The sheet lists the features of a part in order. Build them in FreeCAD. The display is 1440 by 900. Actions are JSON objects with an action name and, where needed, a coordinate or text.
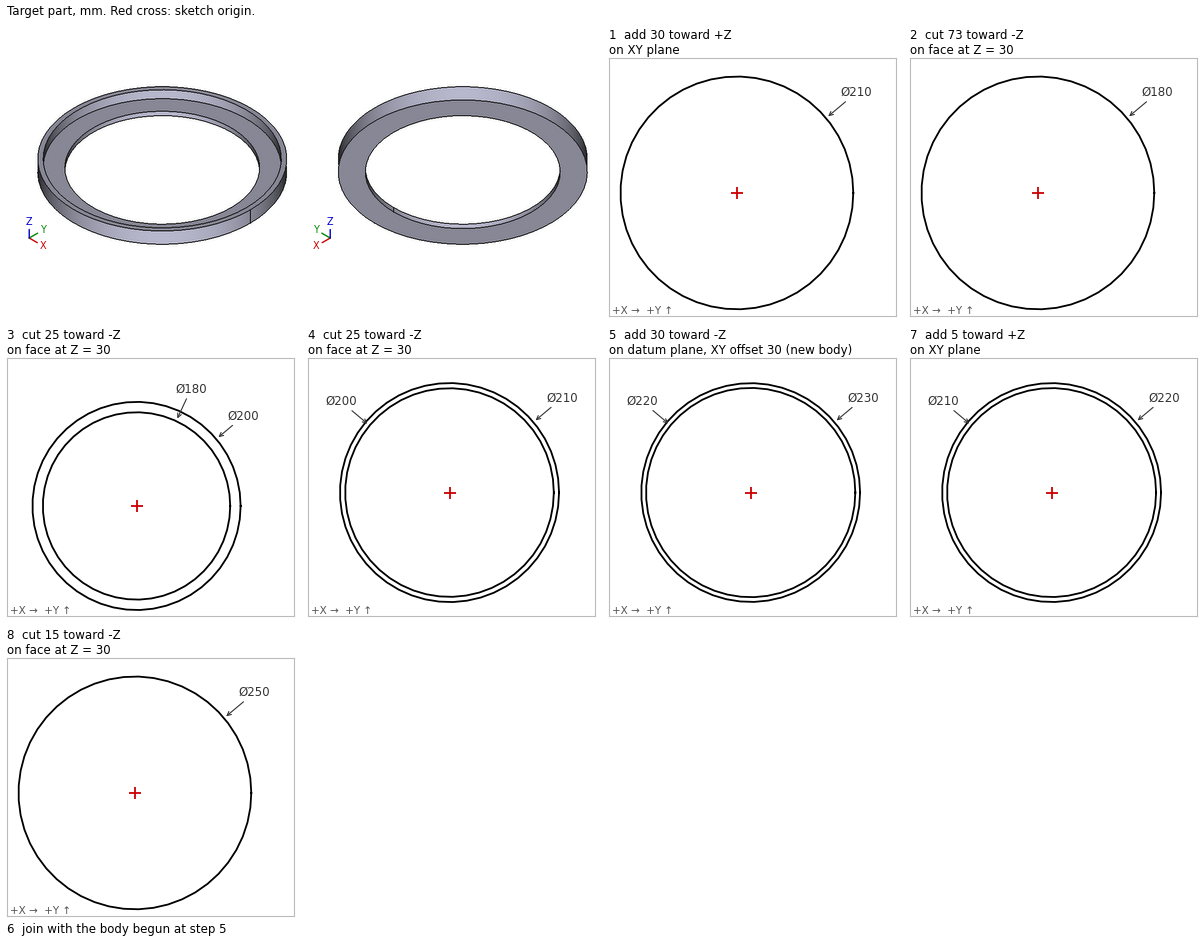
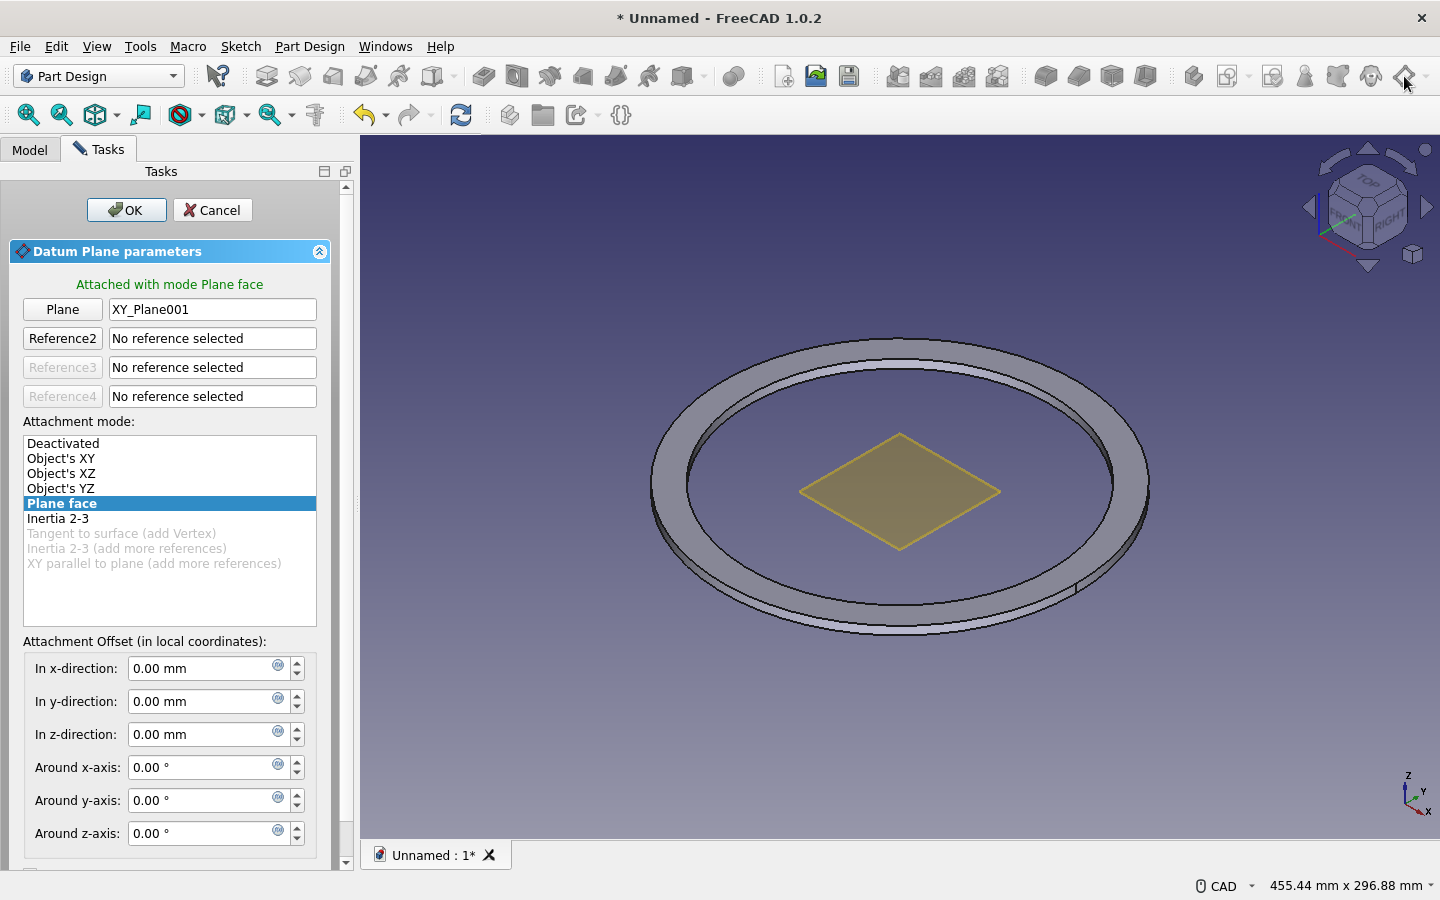
{"action": "triple_click", "coordinate": [210, 734]}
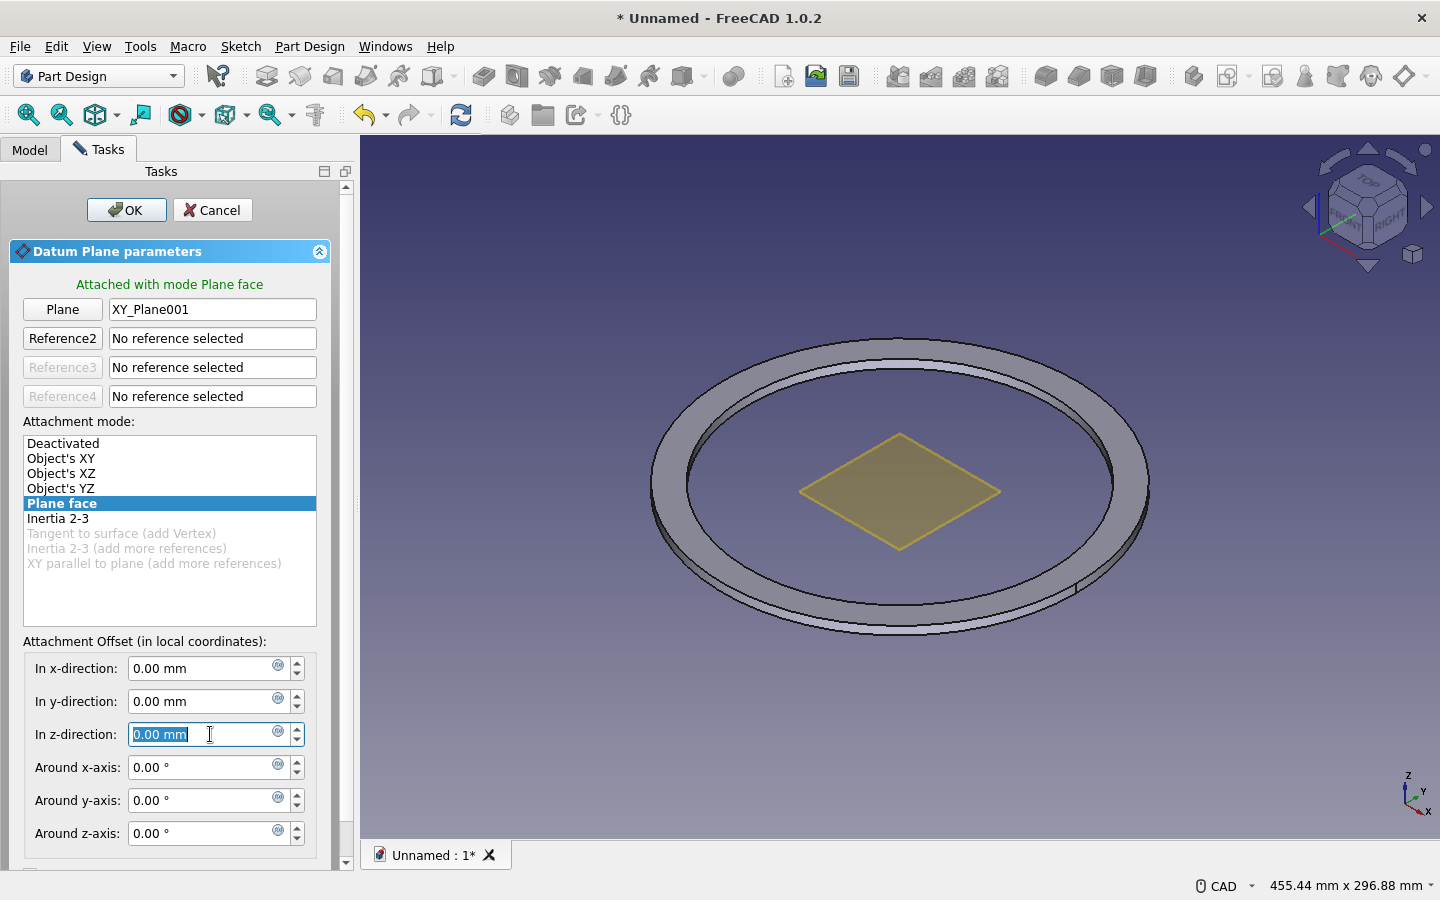
{"action": "type", "text": "30"}
{"action": "key", "text": "Tab"}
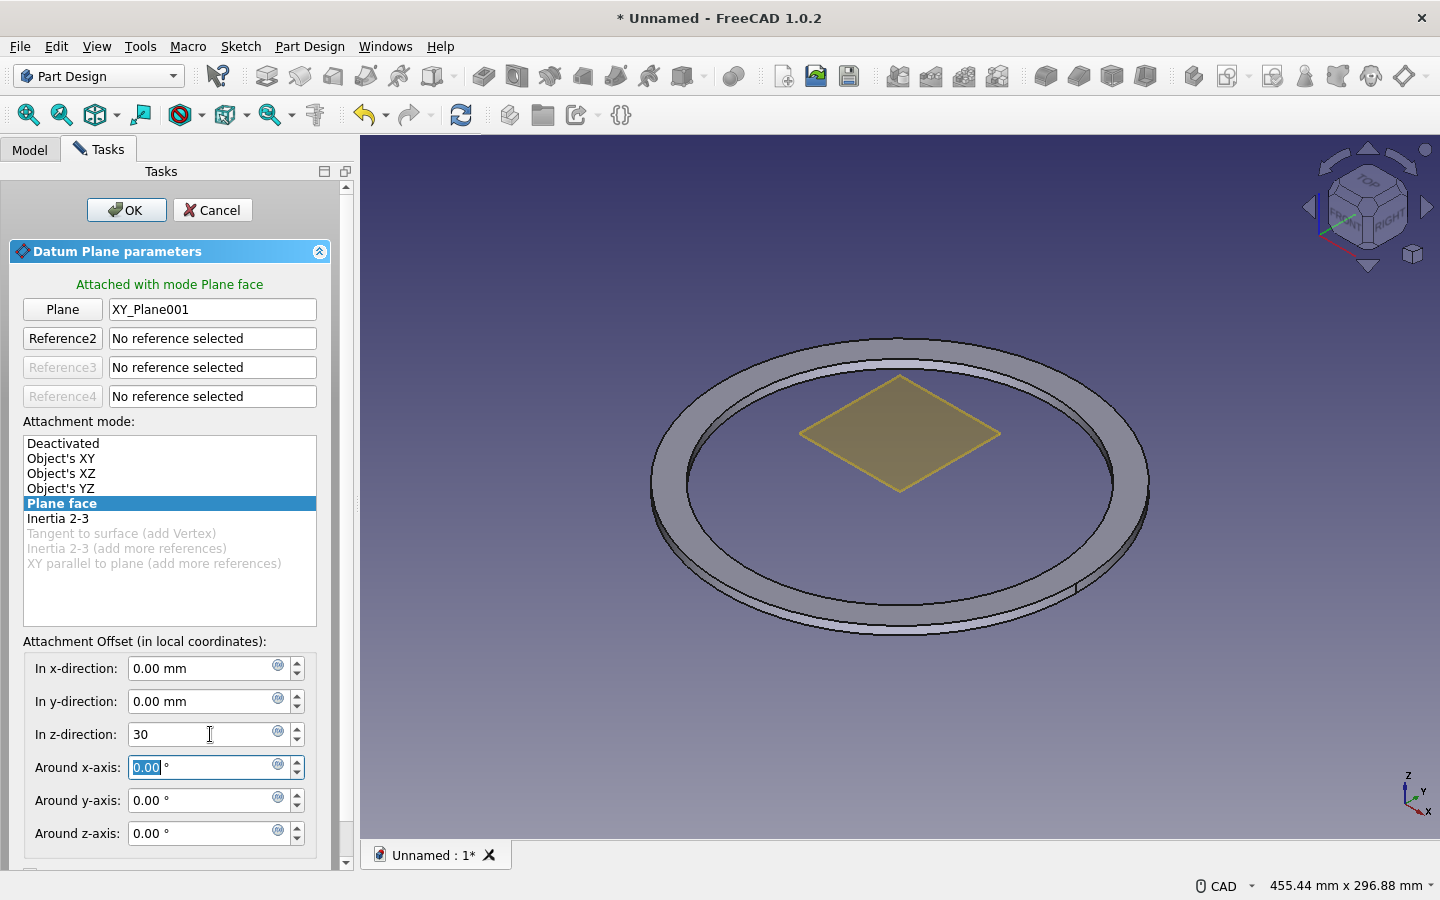
{"action": "left_click", "coordinate": [127, 210]}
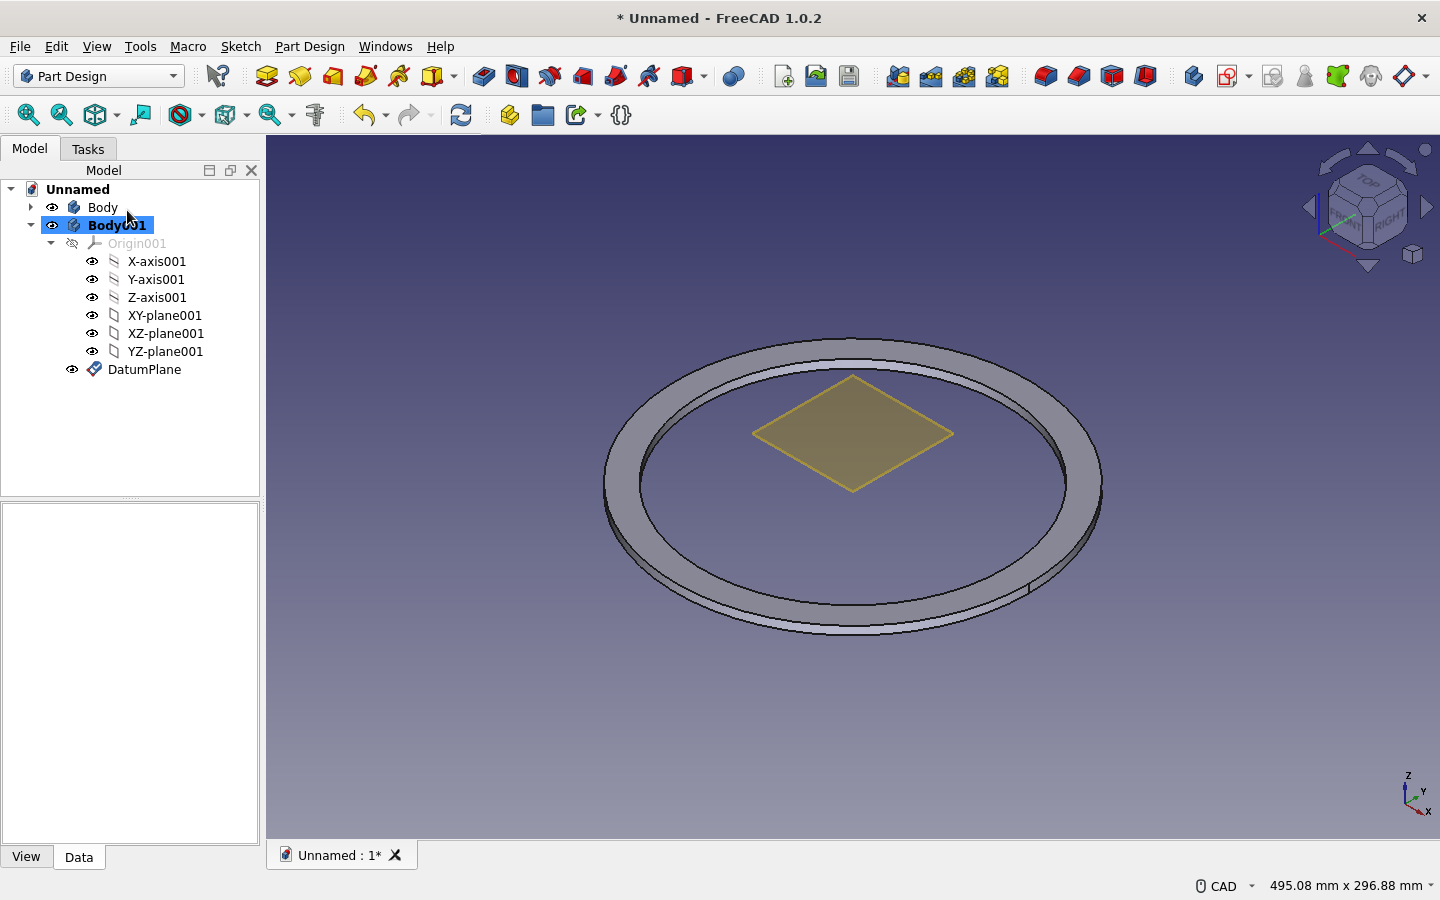
{"action": "left_click", "coordinate": [117, 369]}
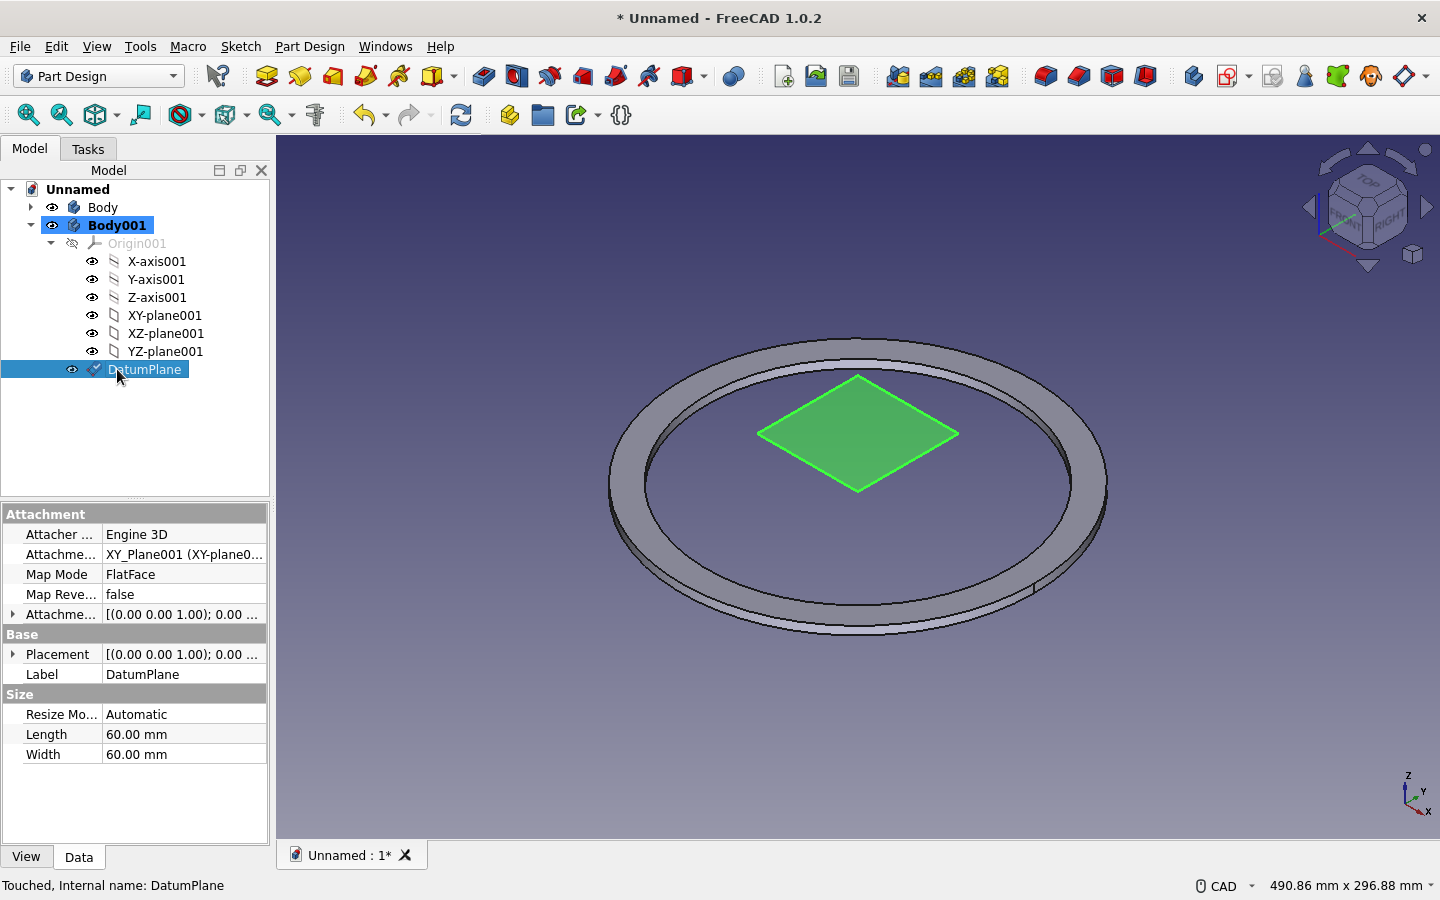
{"action": "left_click", "coordinate": [1226, 76]}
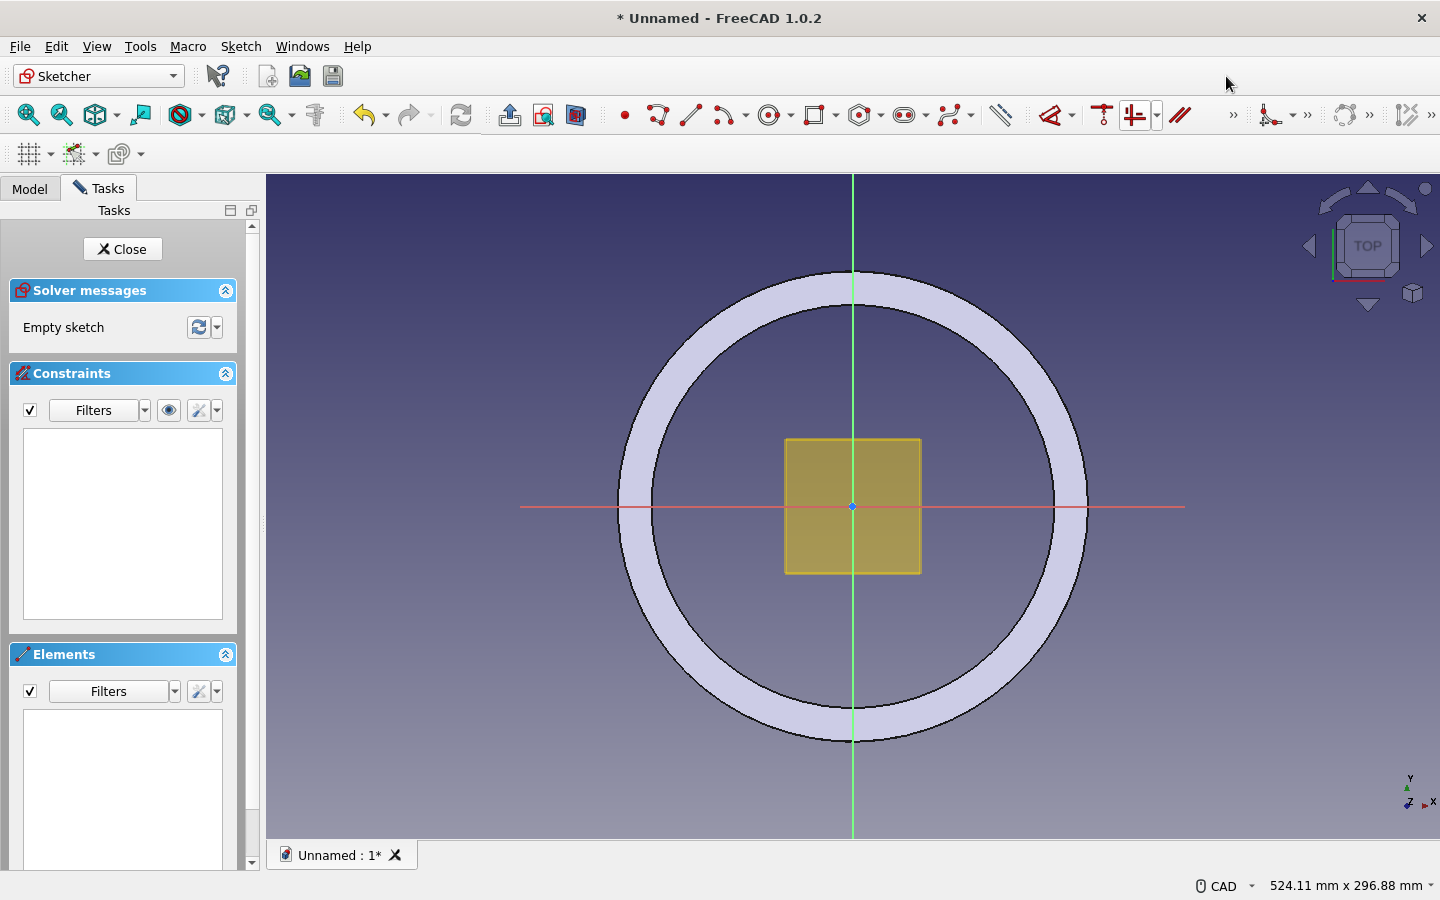
{"action": "left_click", "coordinate": [768, 116]}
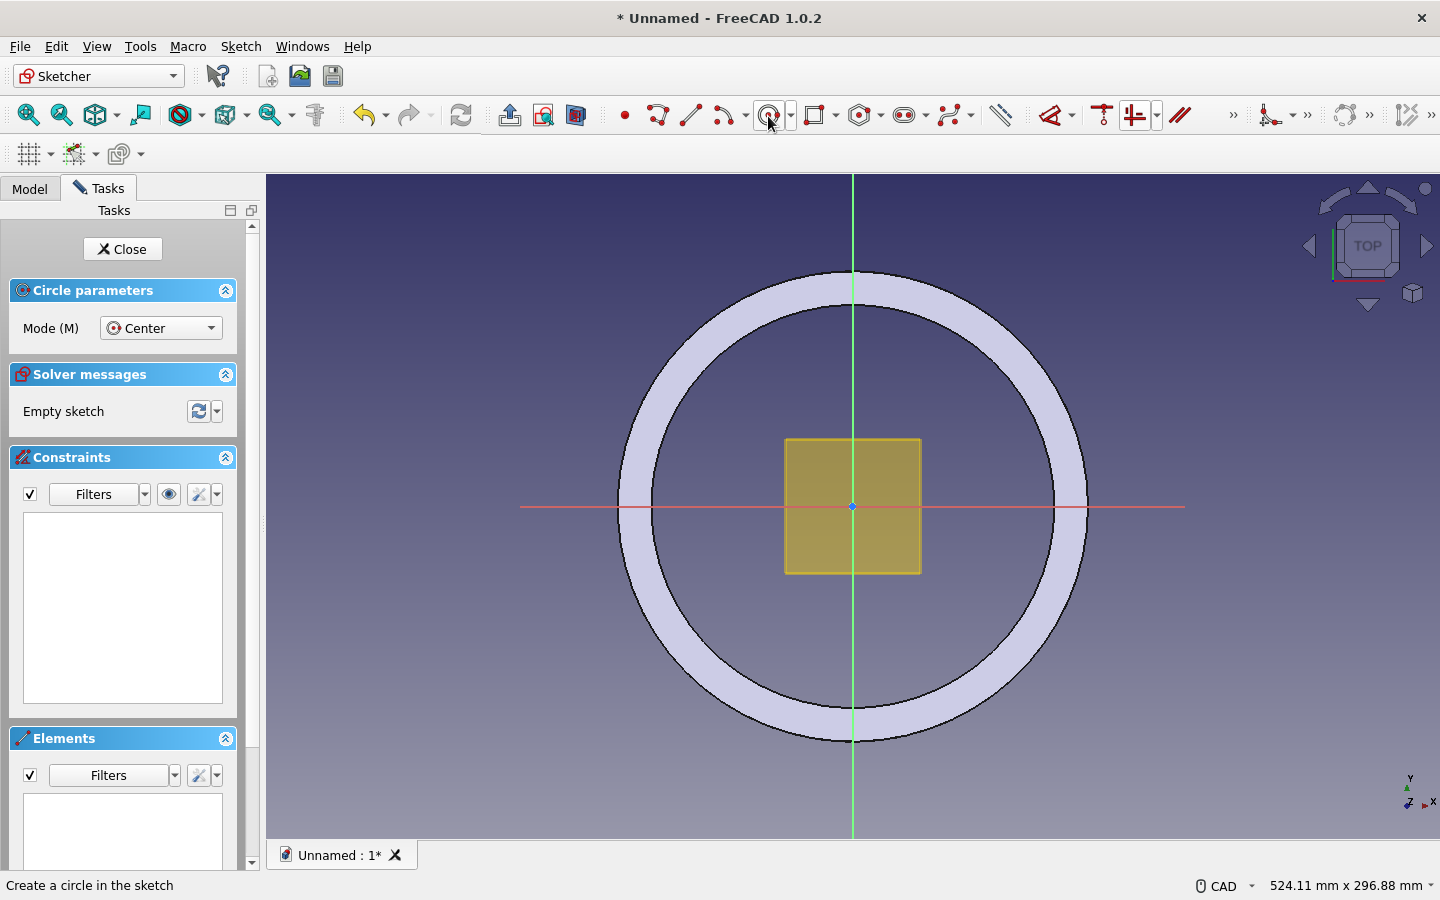
{"action": "left_click", "coordinate": [853, 506]}
{"action": "mouse_move", "coordinate": [1035, 324]}